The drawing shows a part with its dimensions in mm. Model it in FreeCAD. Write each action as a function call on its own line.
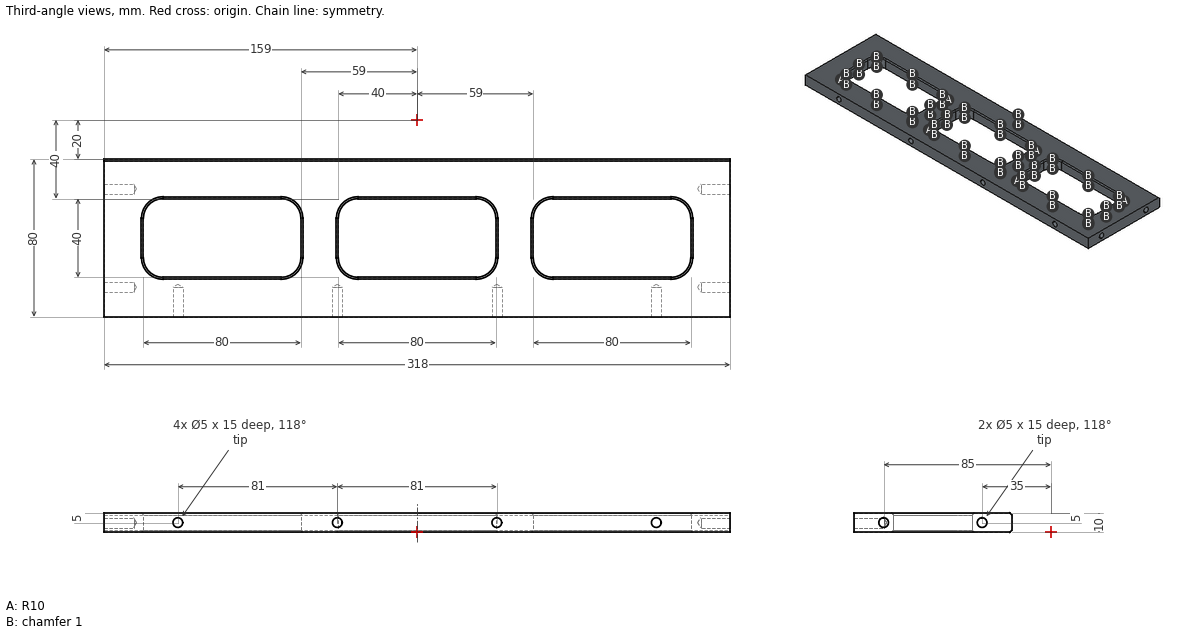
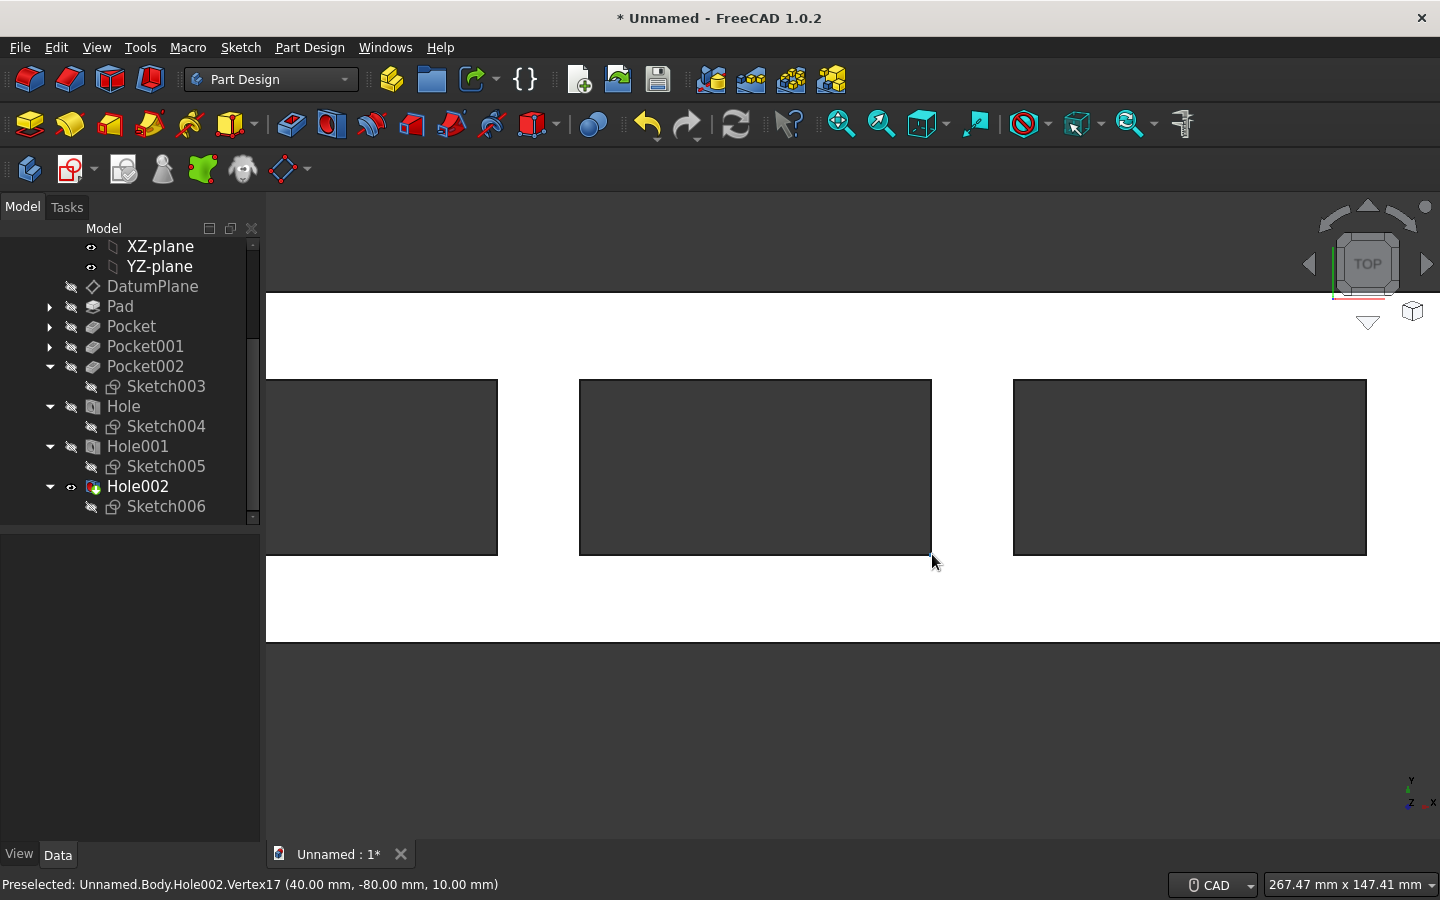
key(v)
key(f)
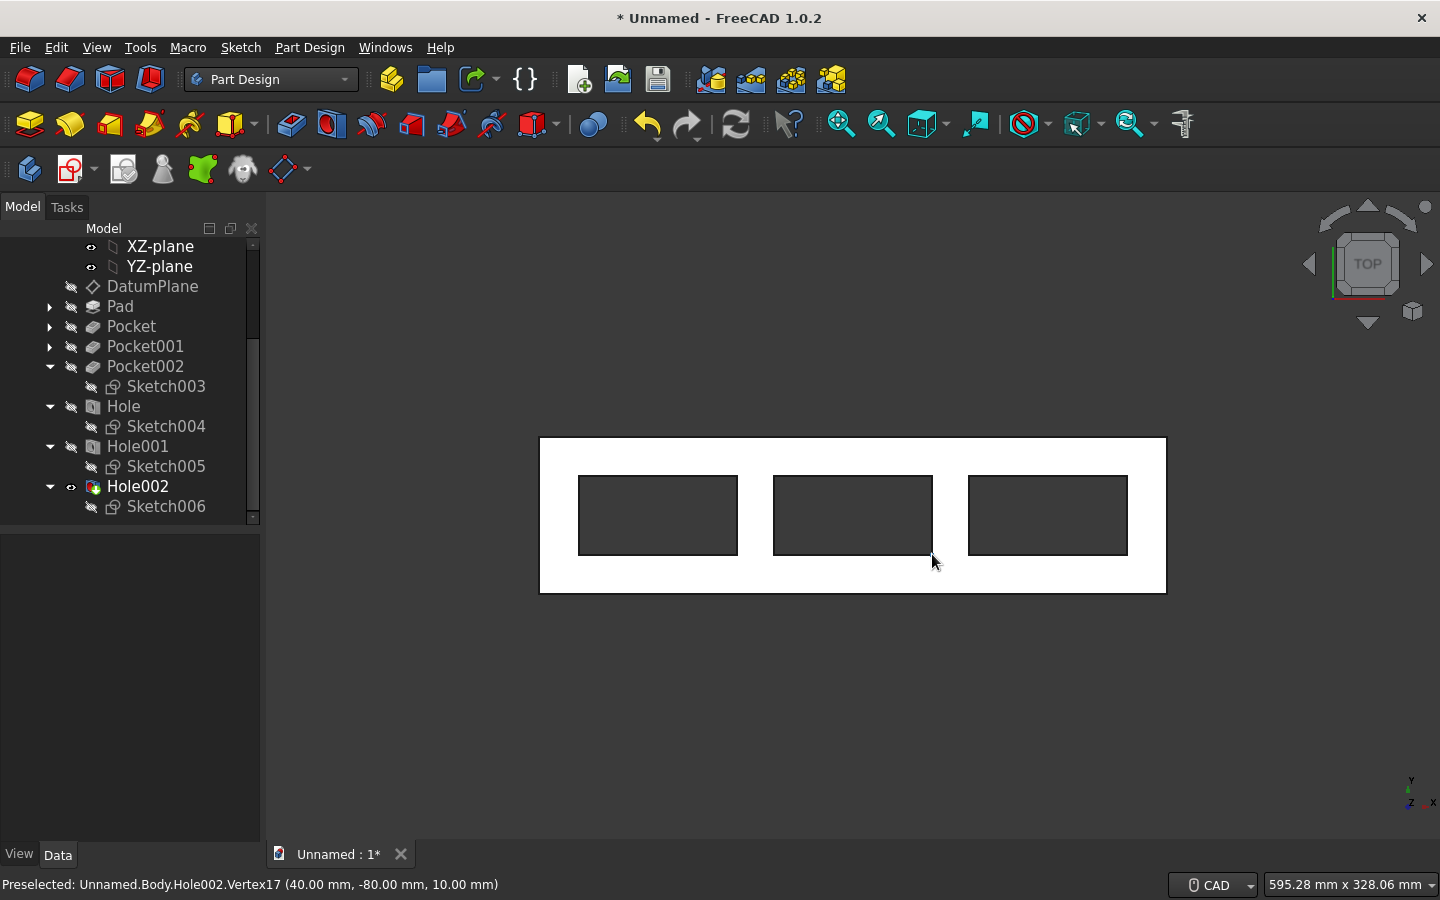
key(1)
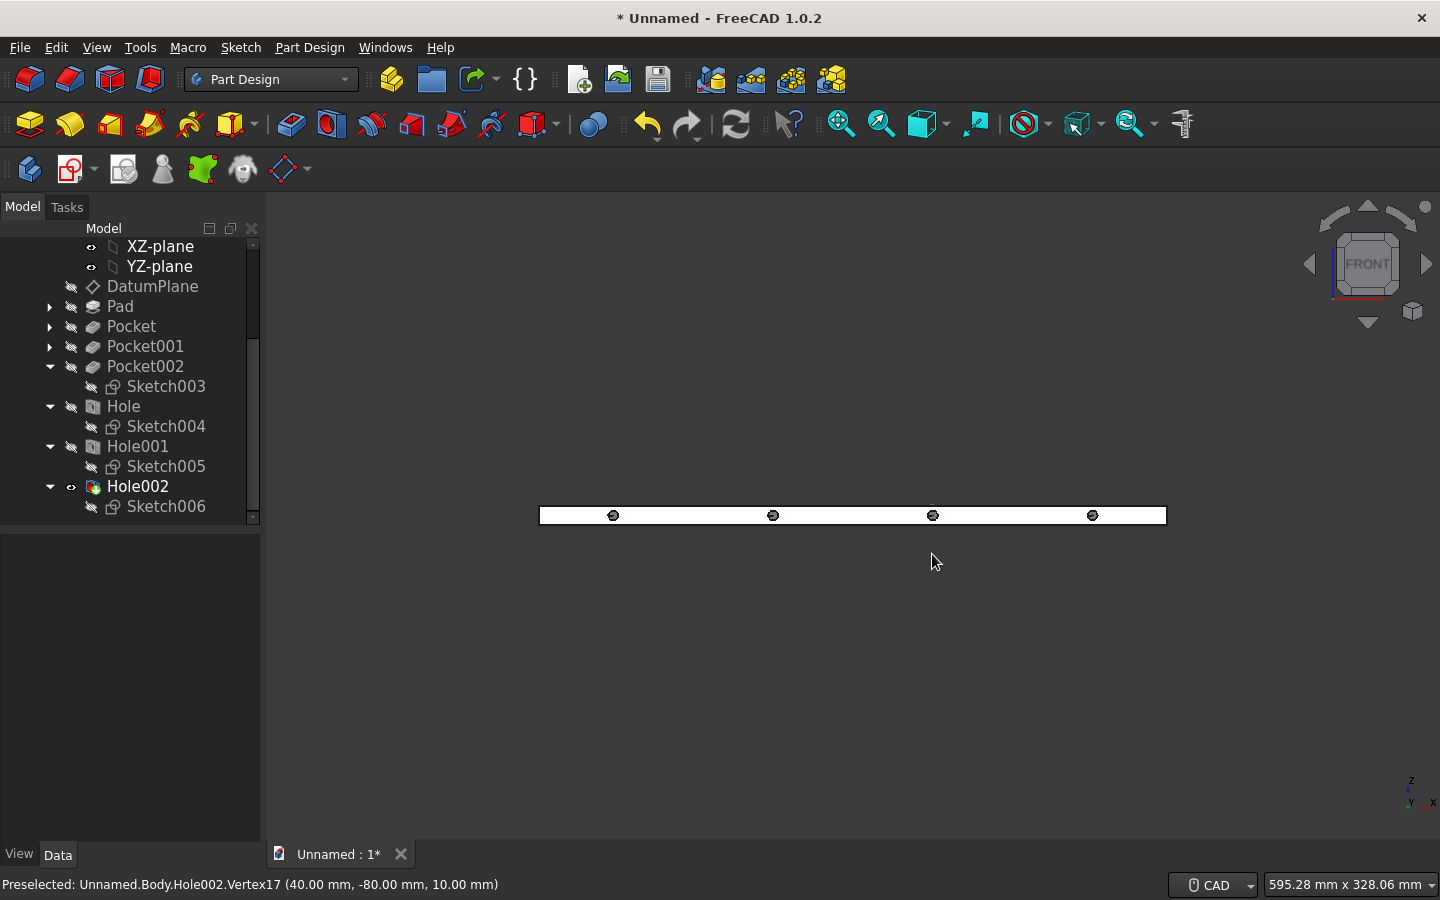
scroll(932, 514, up, 4)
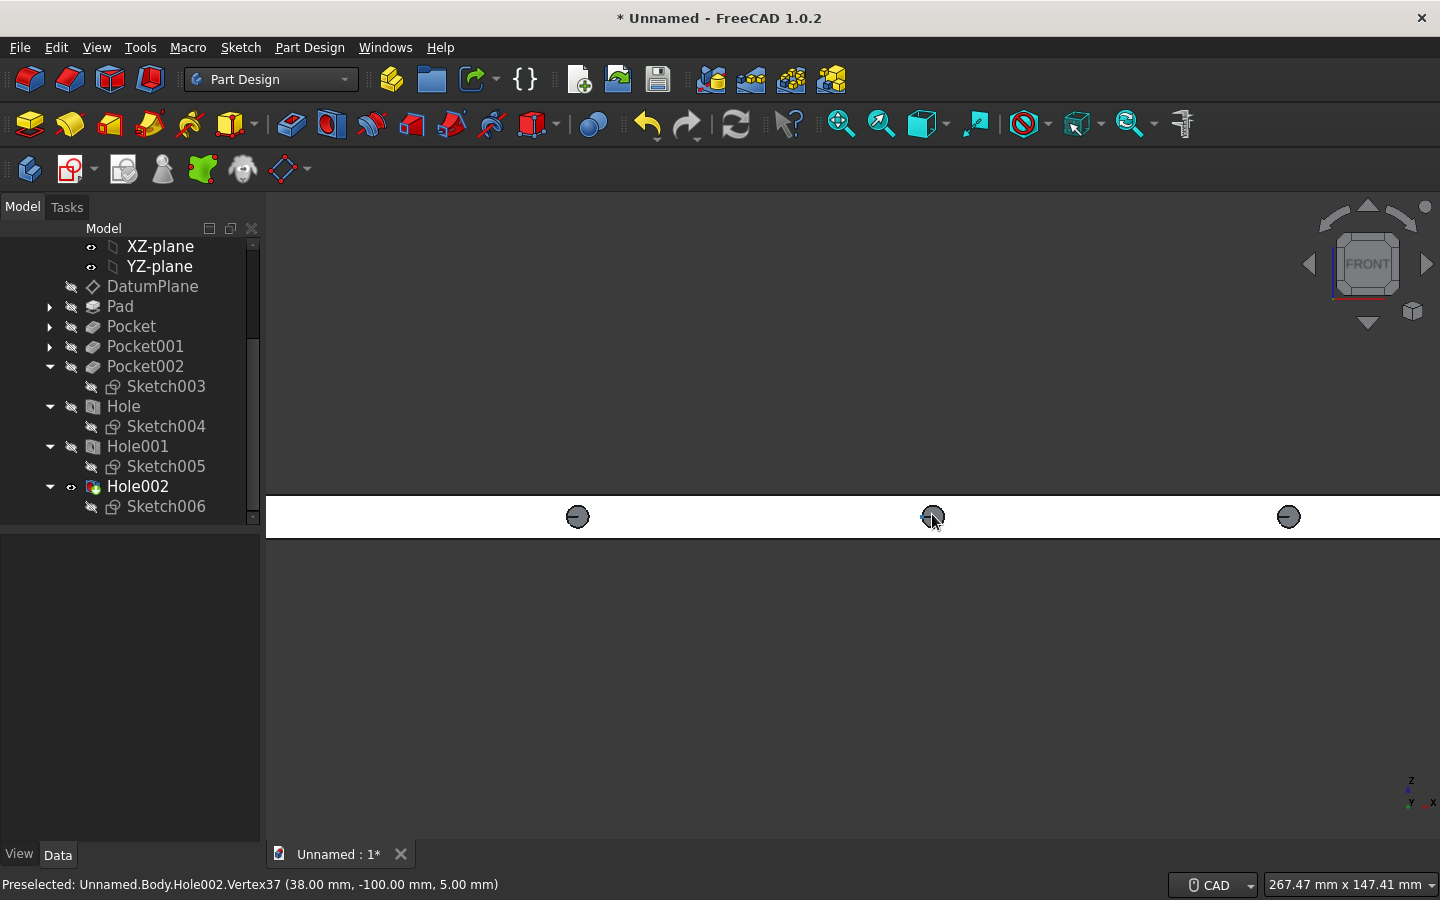
click(842, 124)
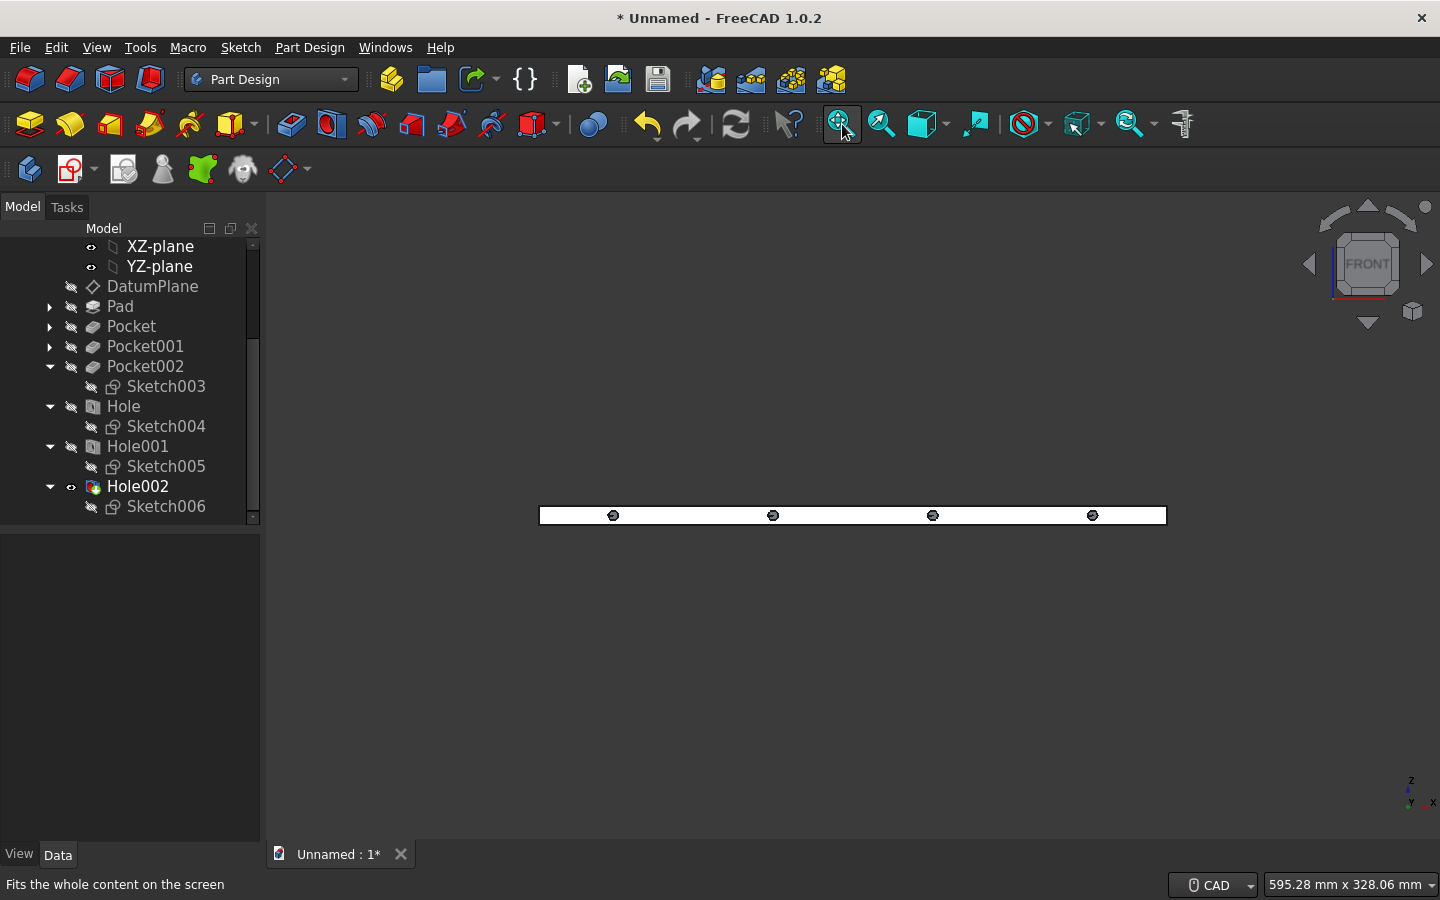
key(3)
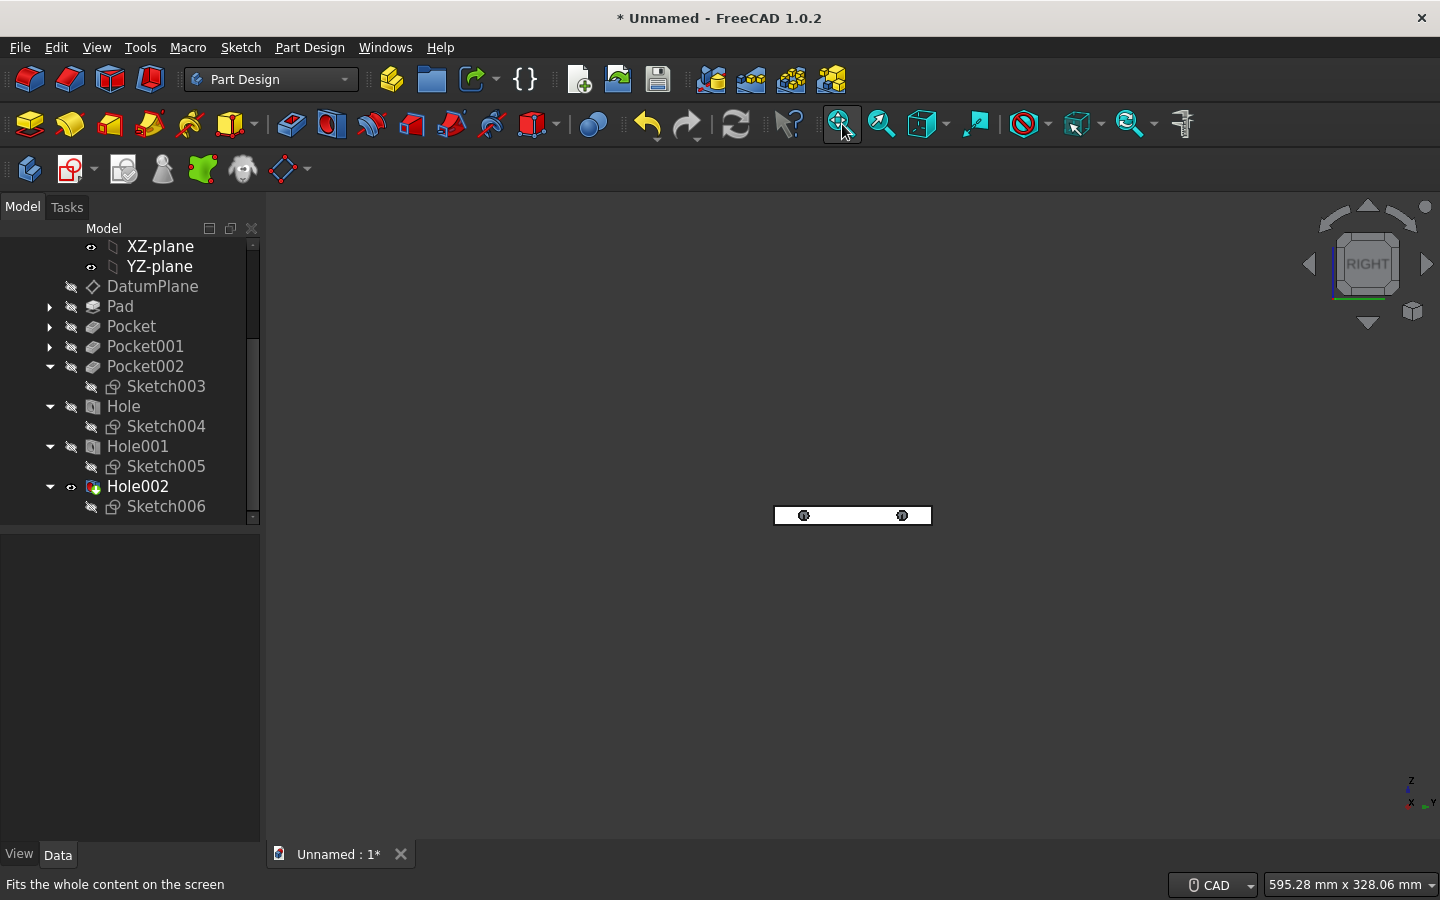
click(842, 124)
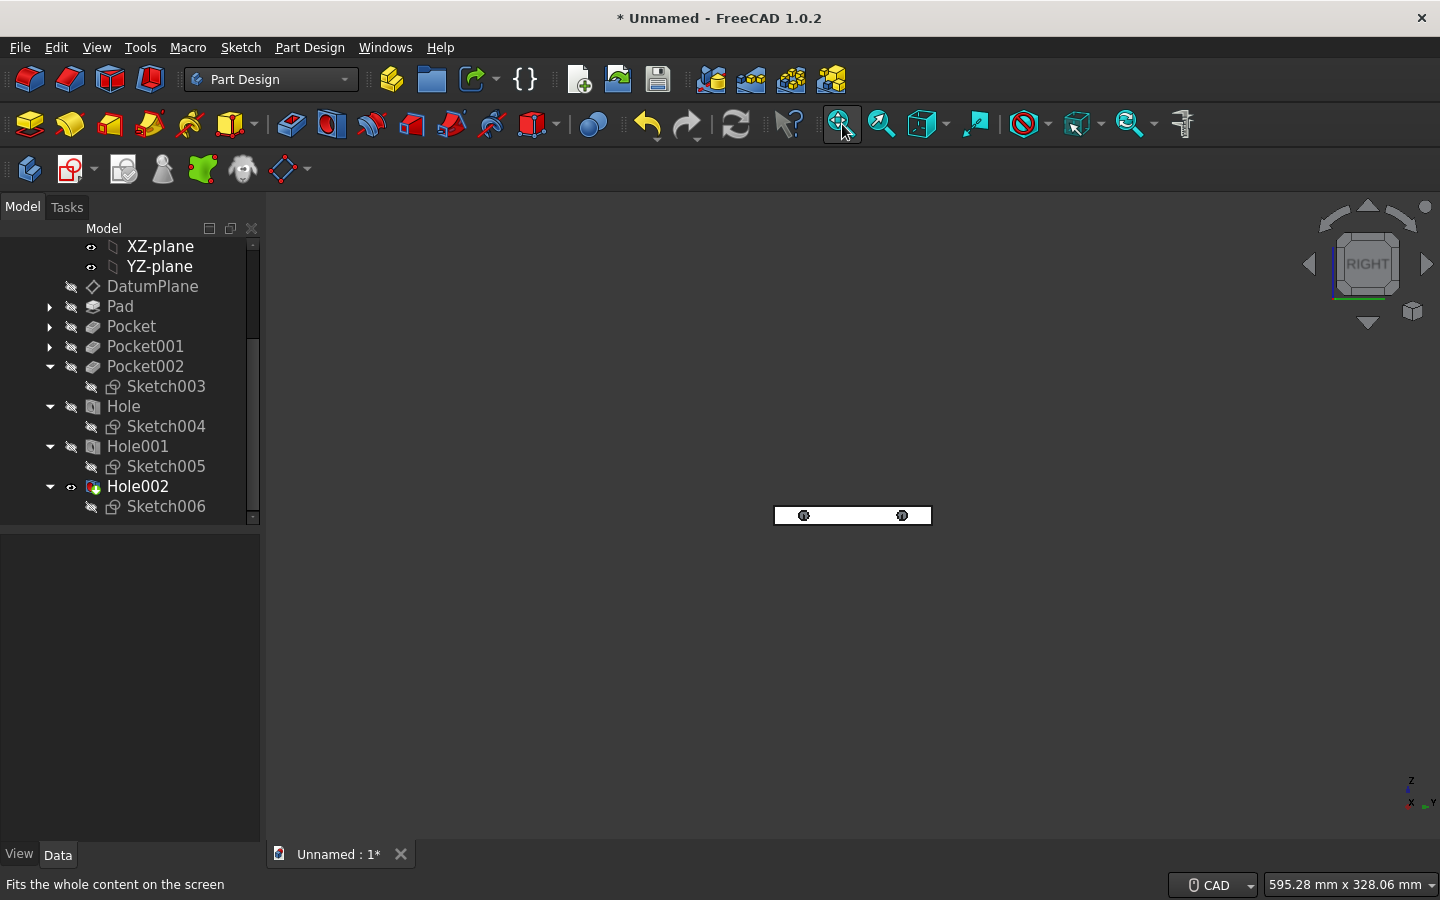
scroll(814, 514, up, 4)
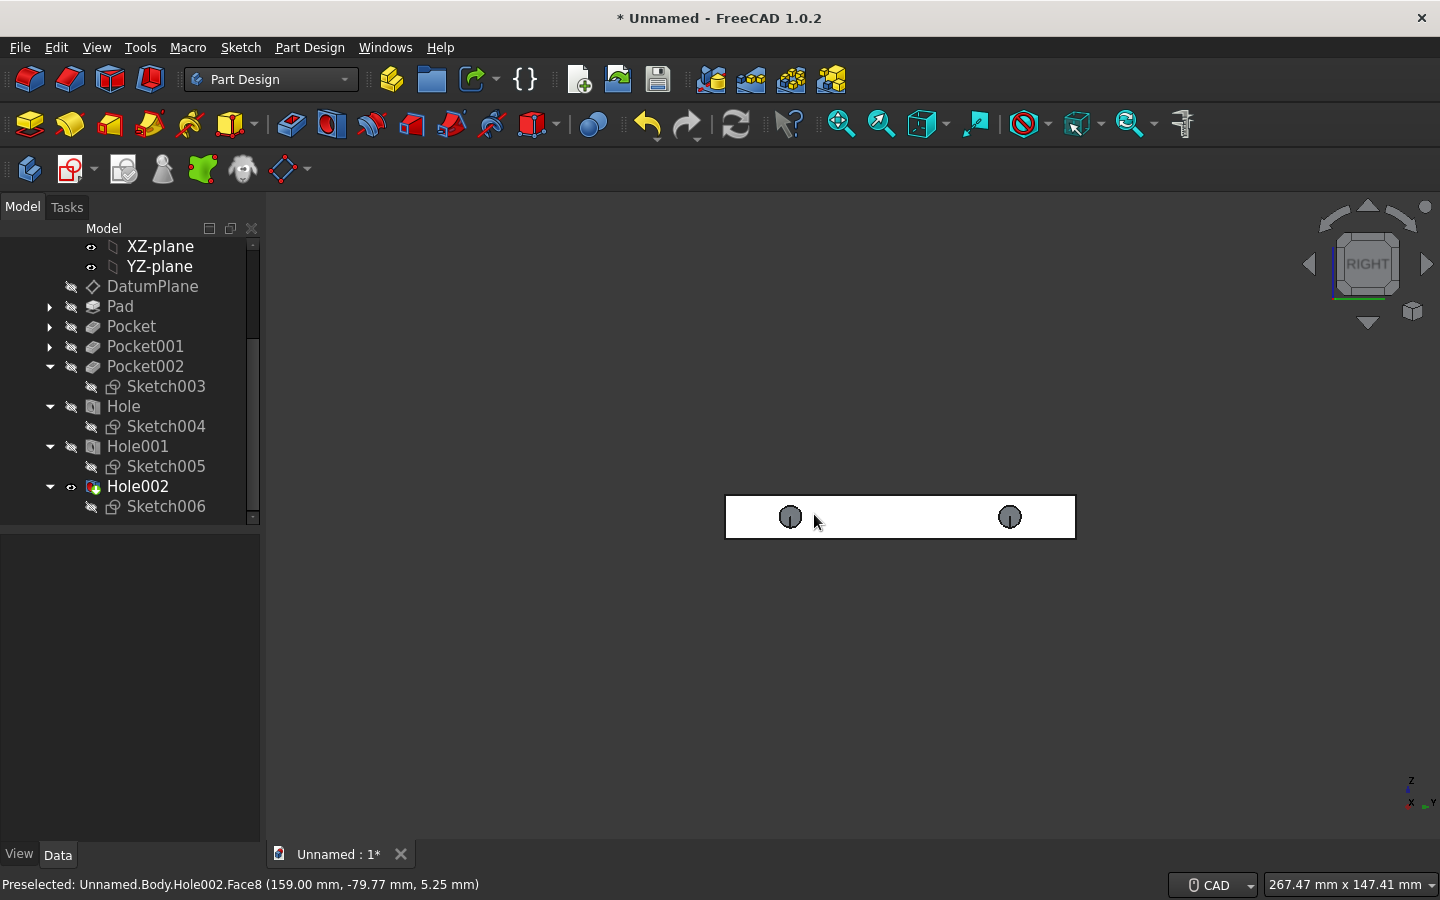
click(842, 124)